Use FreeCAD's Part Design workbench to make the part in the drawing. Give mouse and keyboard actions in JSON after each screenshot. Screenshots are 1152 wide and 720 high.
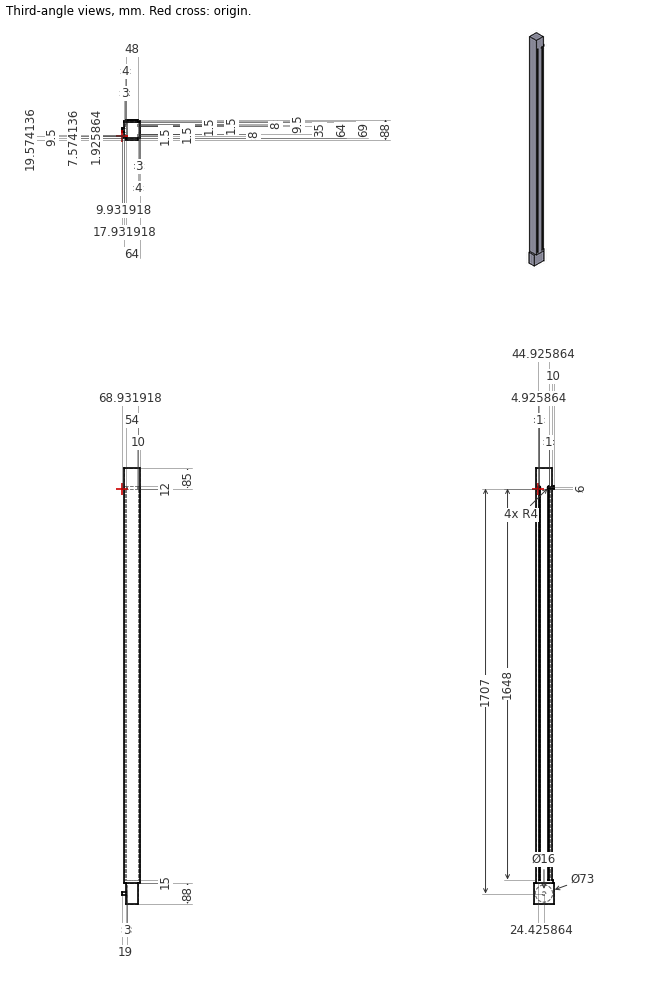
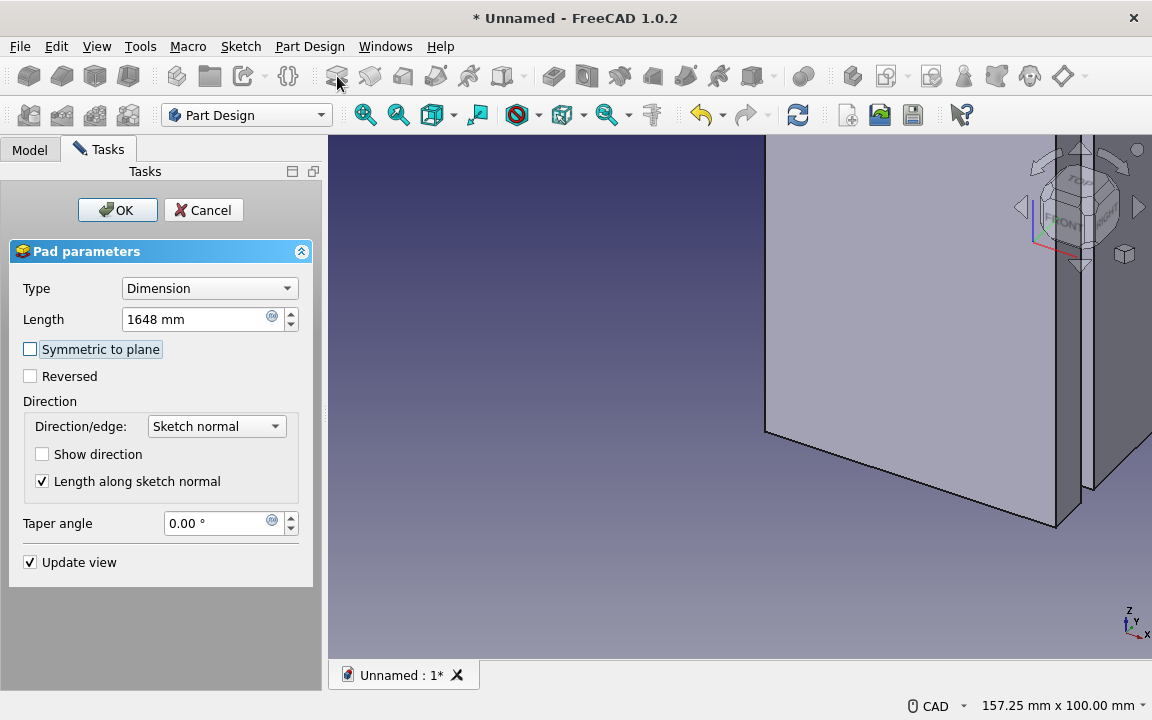
{"action": "left_click", "coordinate": [31, 376]}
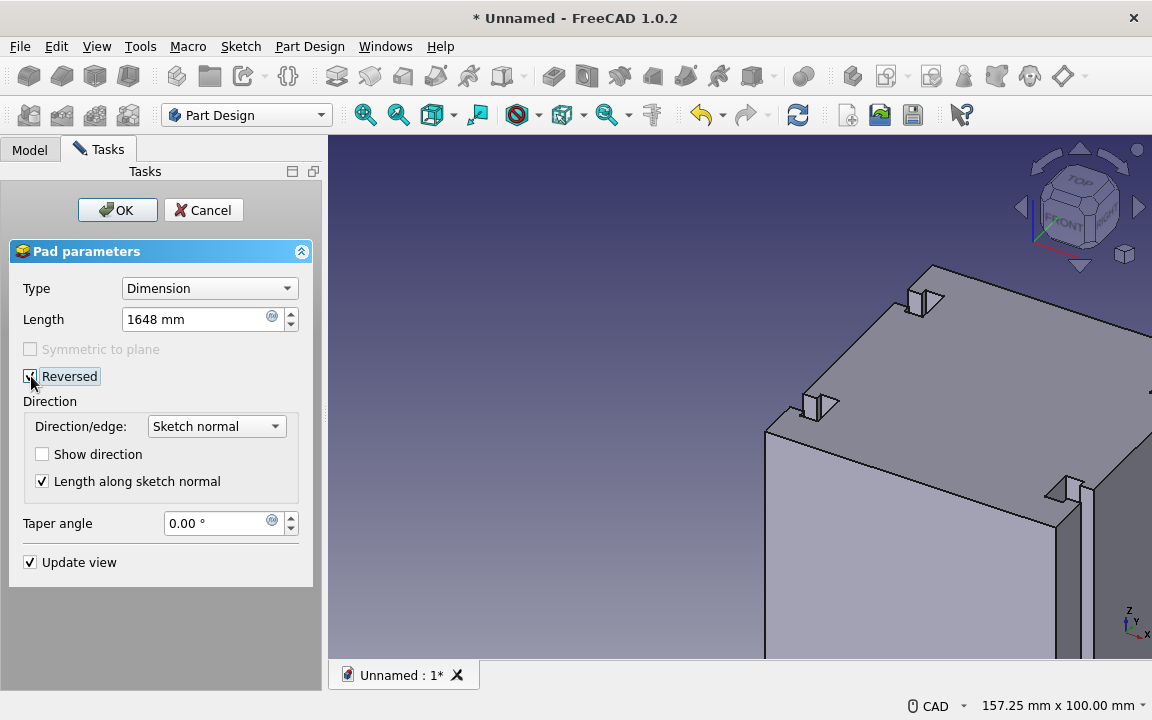
{"action": "left_click", "coordinate": [118, 210]}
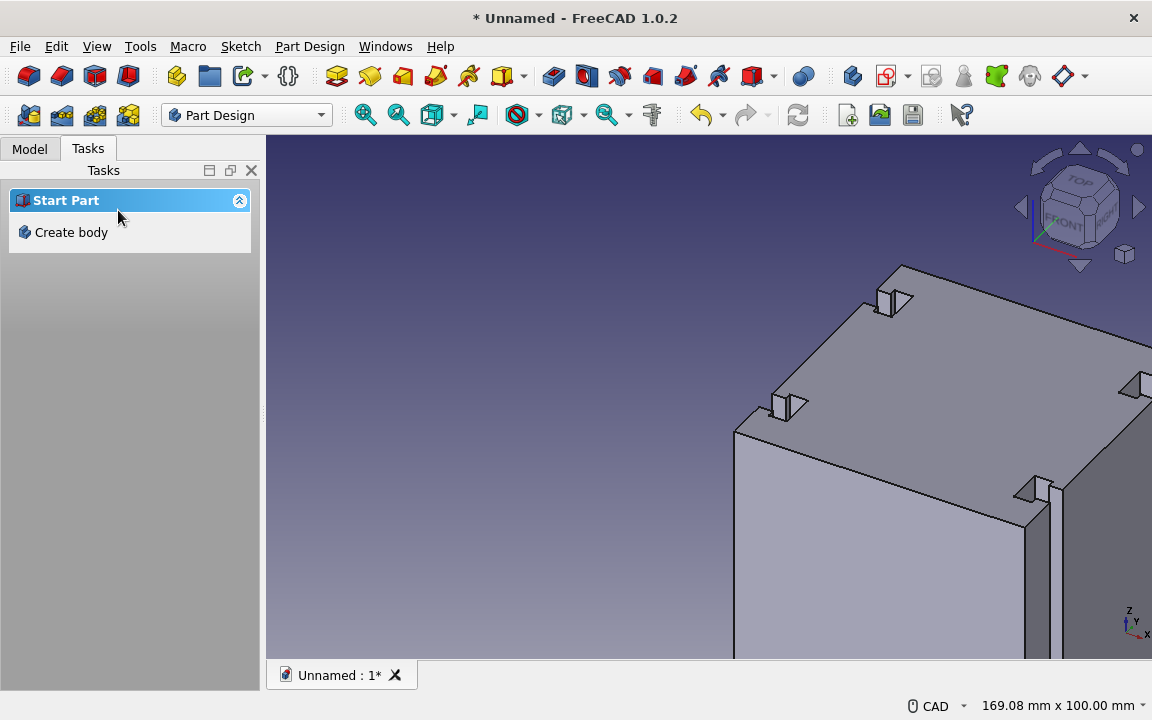
{"action": "left_click", "coordinate": [366, 116]}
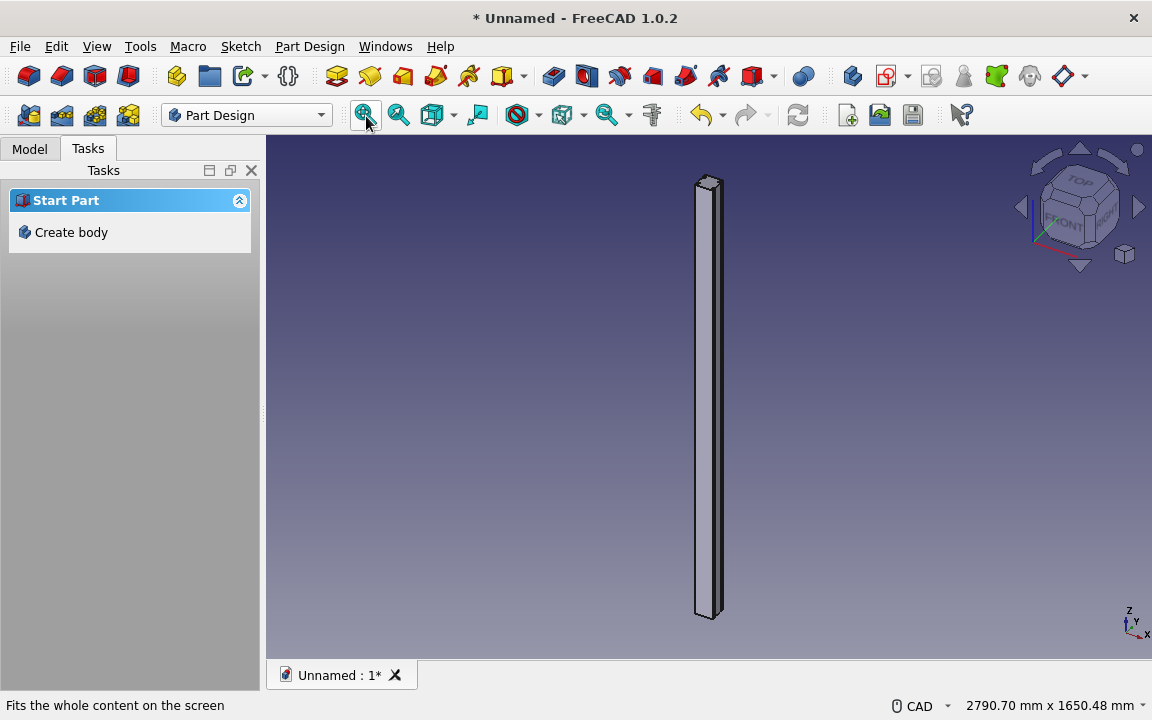
{"action": "left_click", "coordinate": [886, 76]}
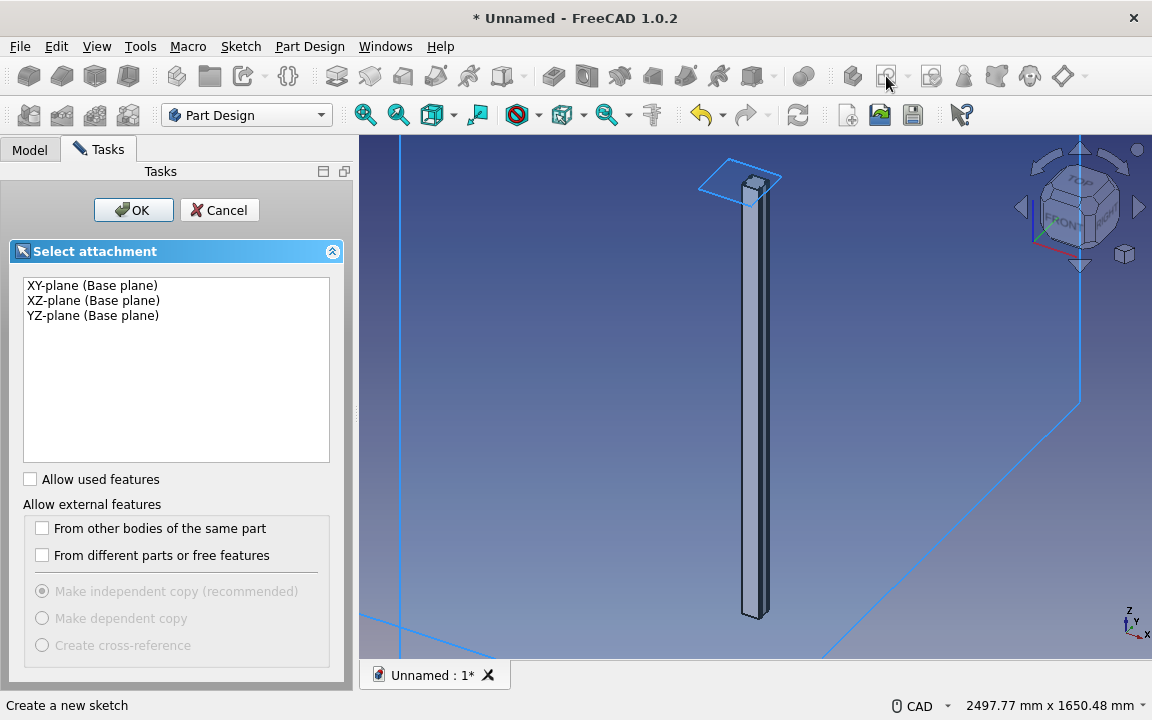
{"action": "left_click", "coordinate": [84, 286]}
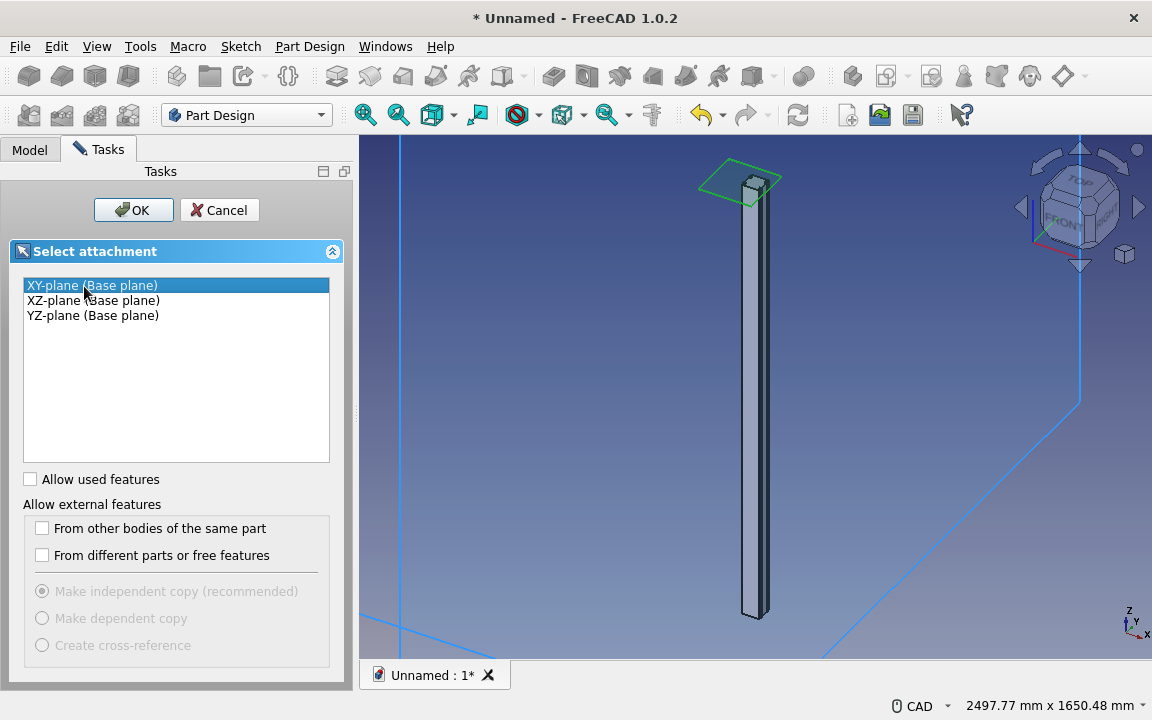
{"action": "left_click", "coordinate": [134, 210]}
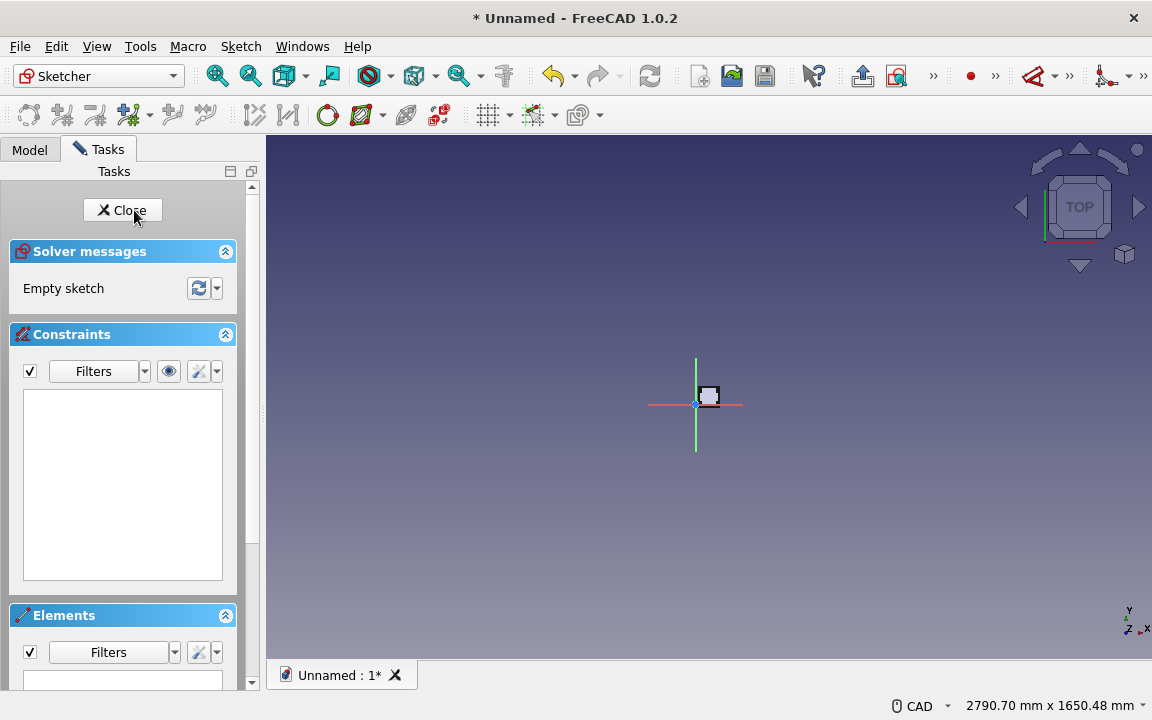
{"action": "scroll", "coordinate": [712, 397], "scroll_direction": "up", "scroll_amount": 14}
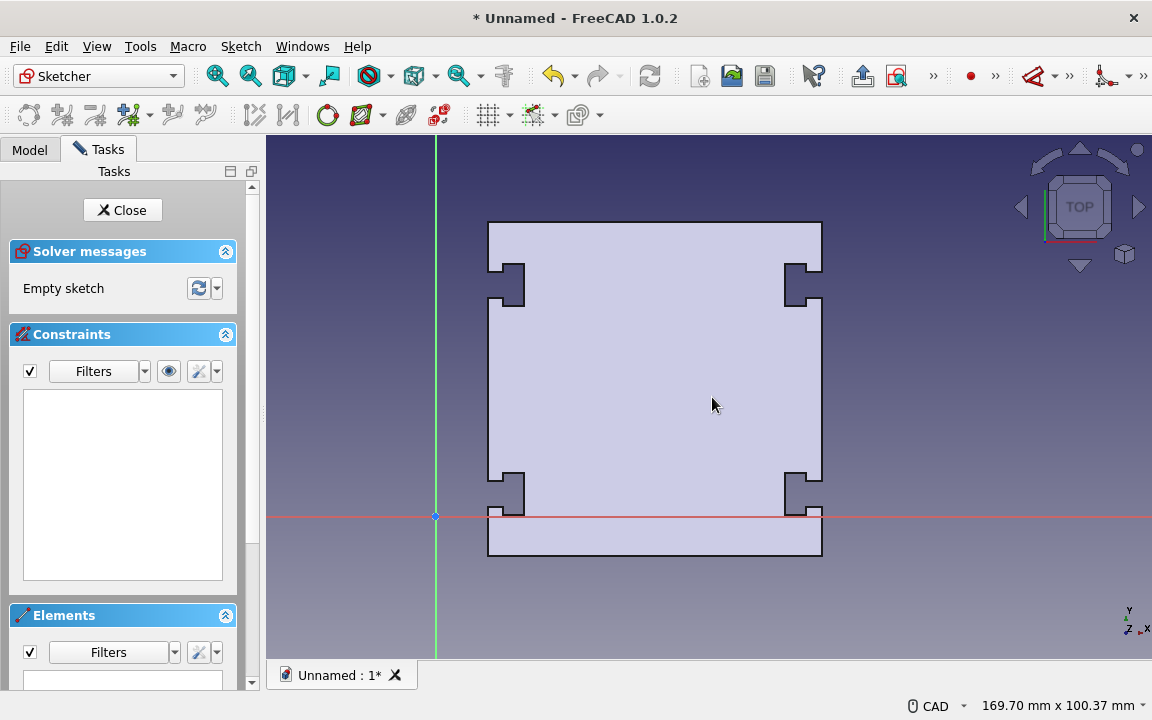
{"action": "key", "text": "g r"}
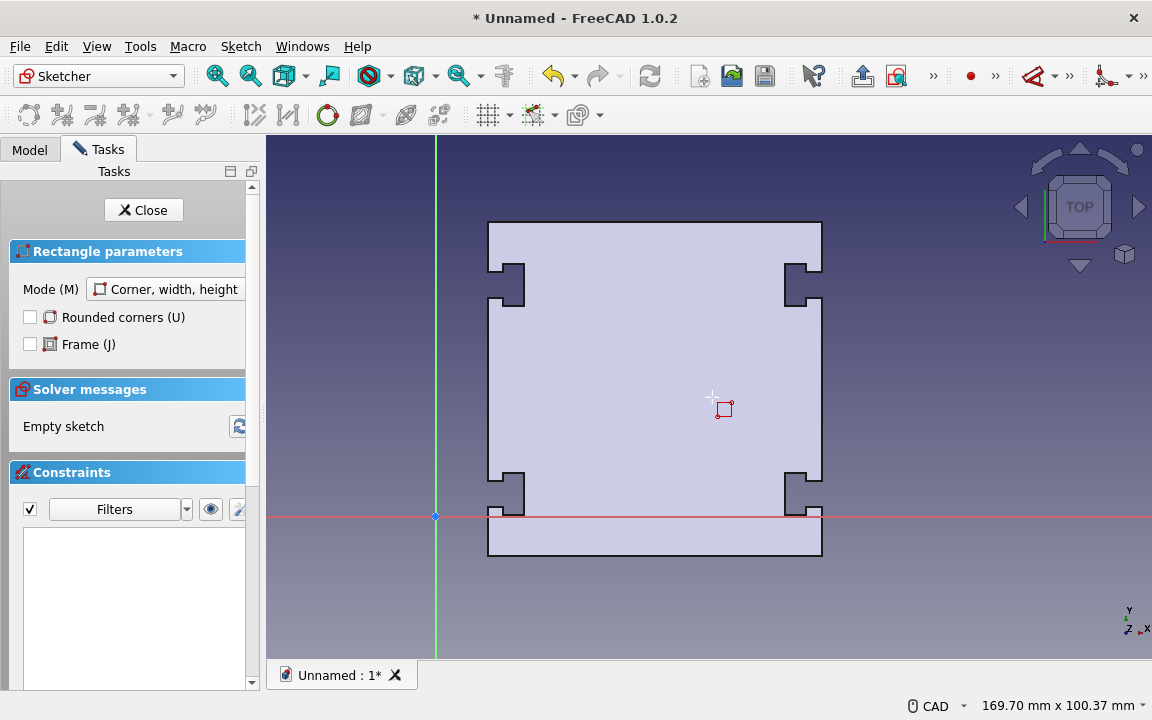
{"action": "left_click", "coordinate": [488, 222]}
{"action": "mouse_move", "coordinate": [822, 556]}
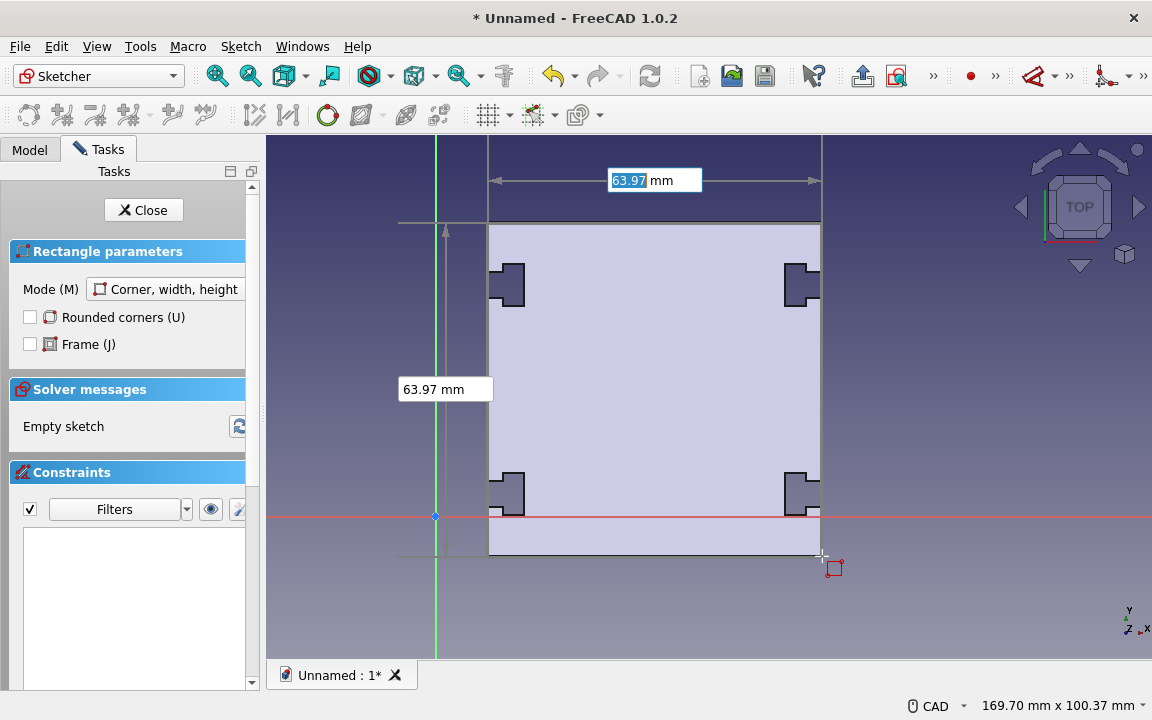
{"action": "type", "text": "64"}
{"action": "key", "text": "Tab"}
{"action": "type", "text": "64"}
{"action": "key", "text": "Return"}
{"action": "key", "text": "Escape"}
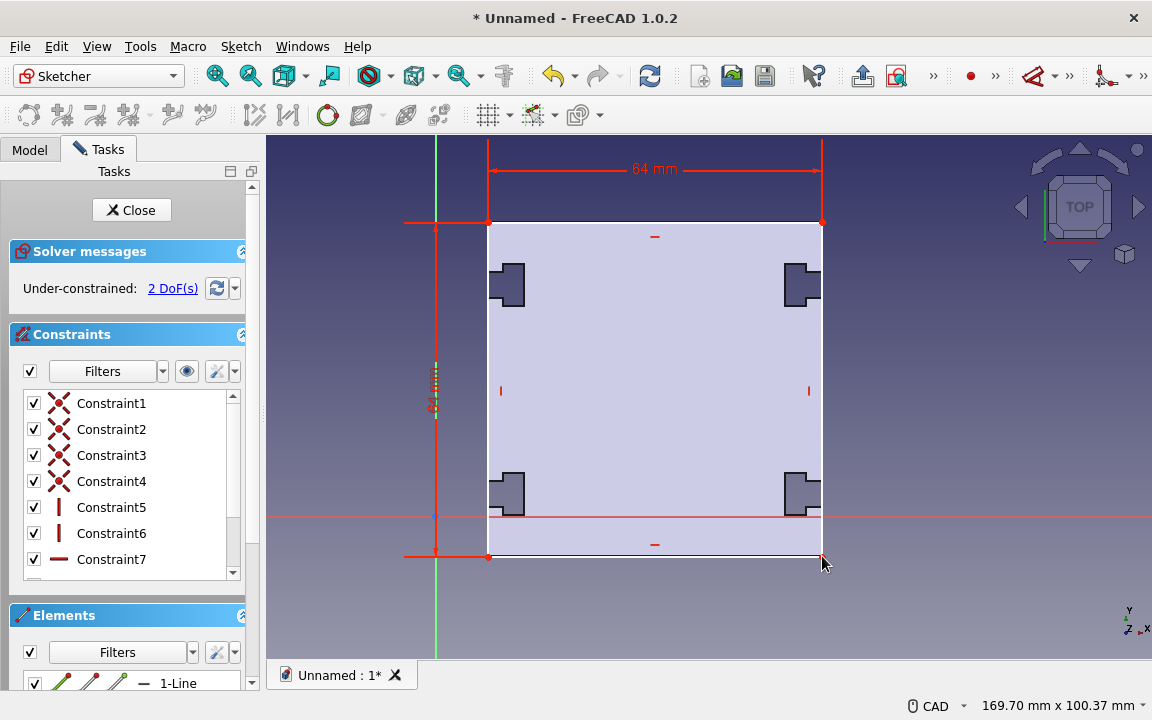
{"action": "left_click", "coordinate": [1032, 76]}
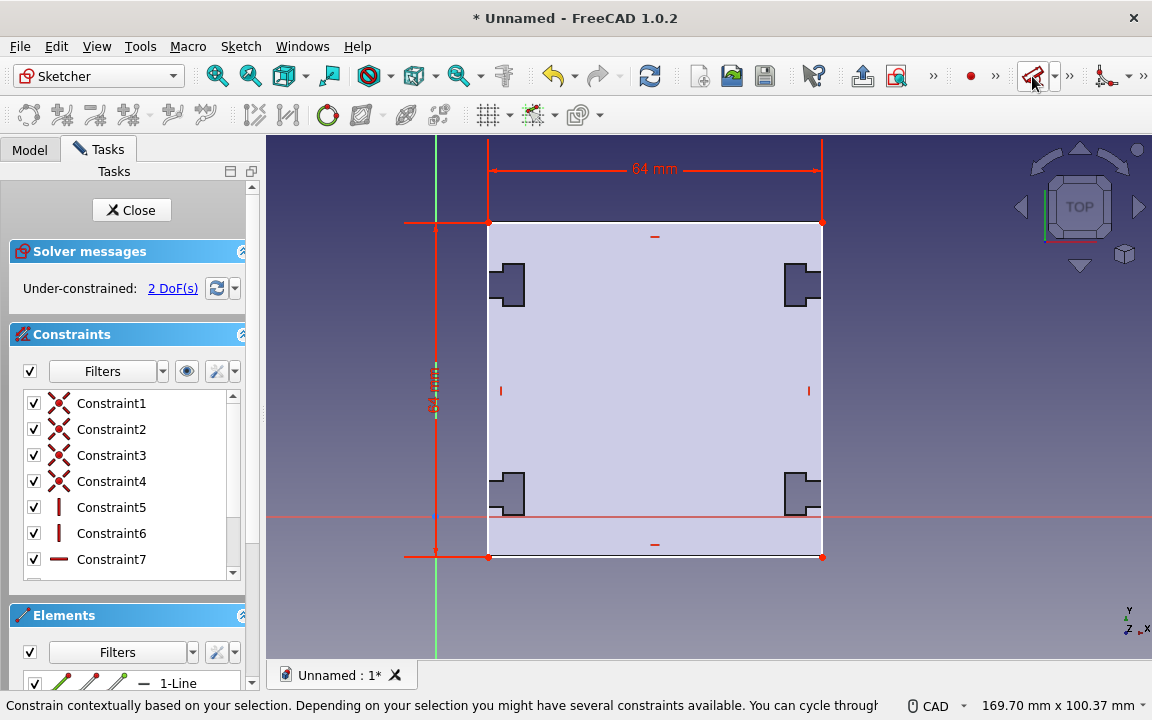
{"action": "left_click", "coordinate": [488, 223]}
{"action": "left_click", "coordinate": [462, 189]}